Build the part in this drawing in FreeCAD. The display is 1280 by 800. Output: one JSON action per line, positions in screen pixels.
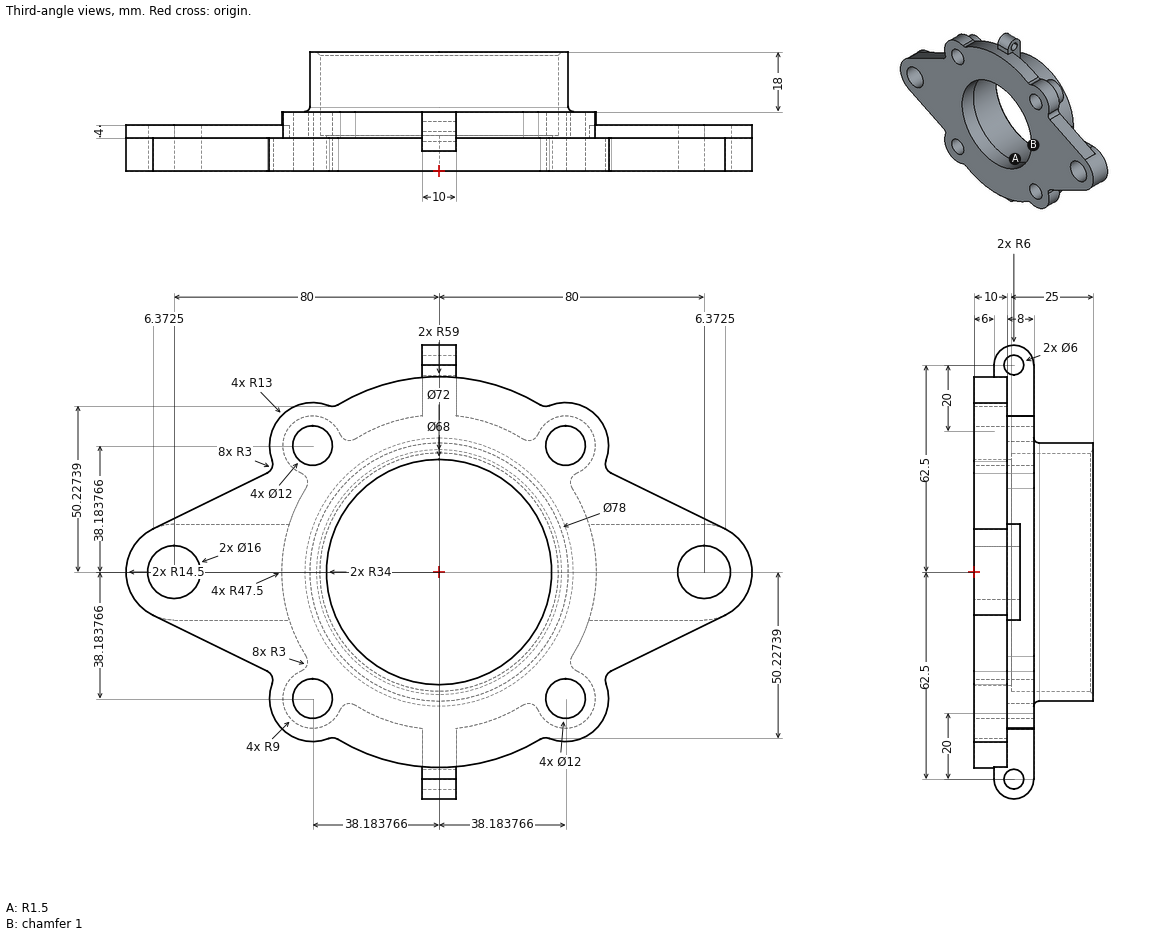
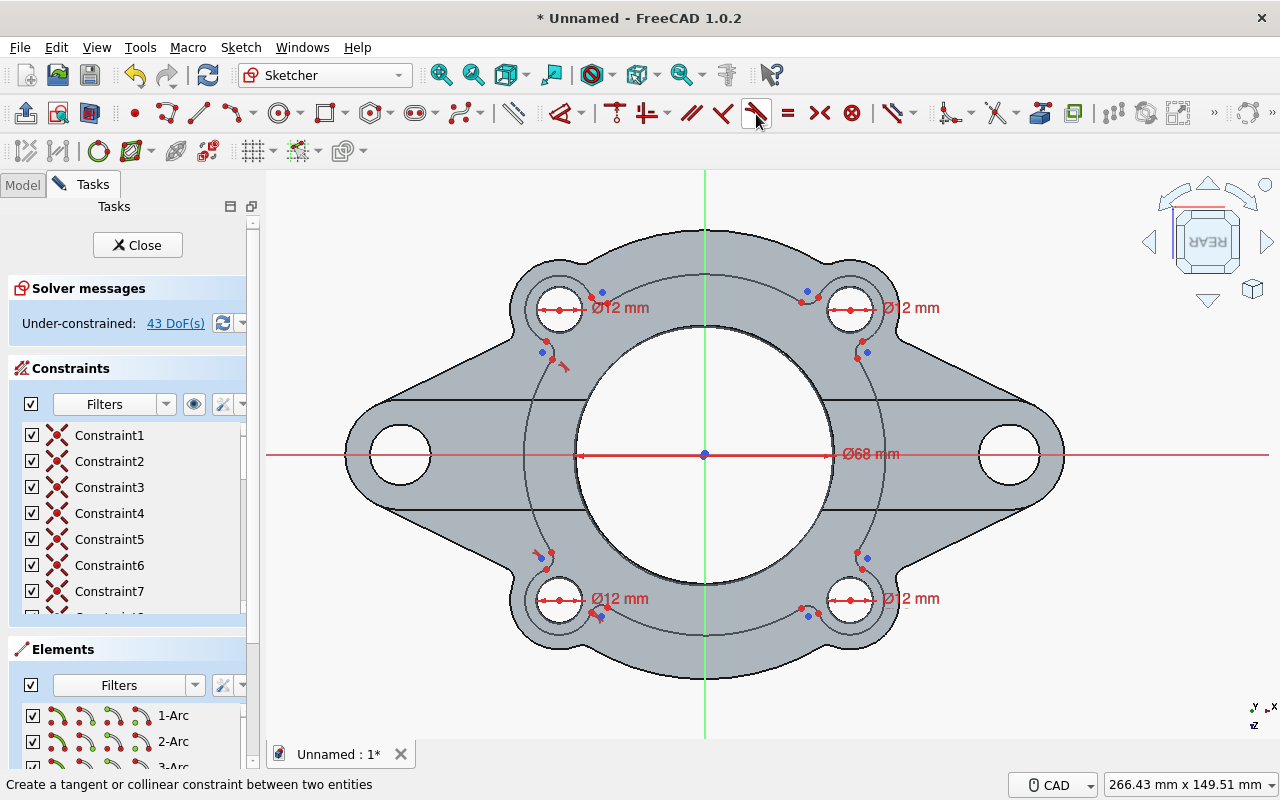
{"action": "left_click", "coordinate": [664, 631]}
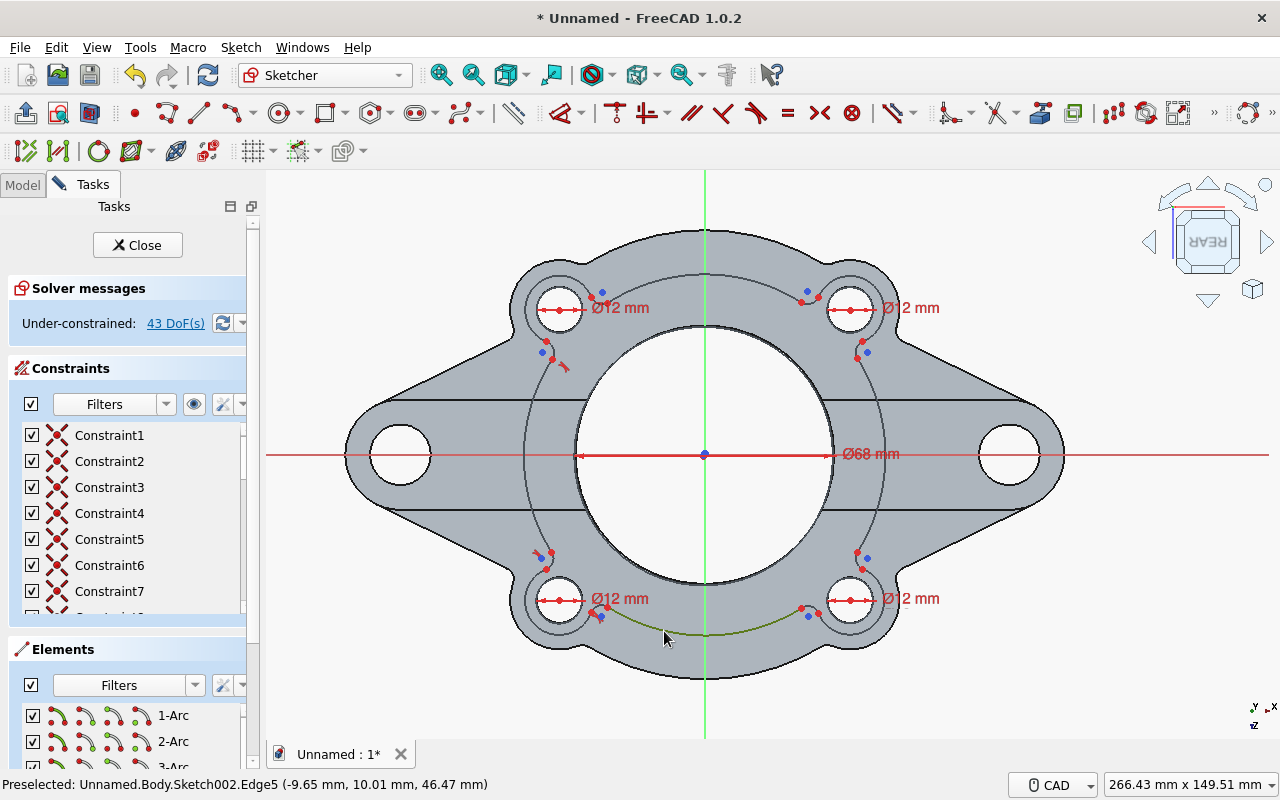
{"action": "scroll", "coordinate": [812, 607], "scroll_direction": "up", "scroll_amount": 2}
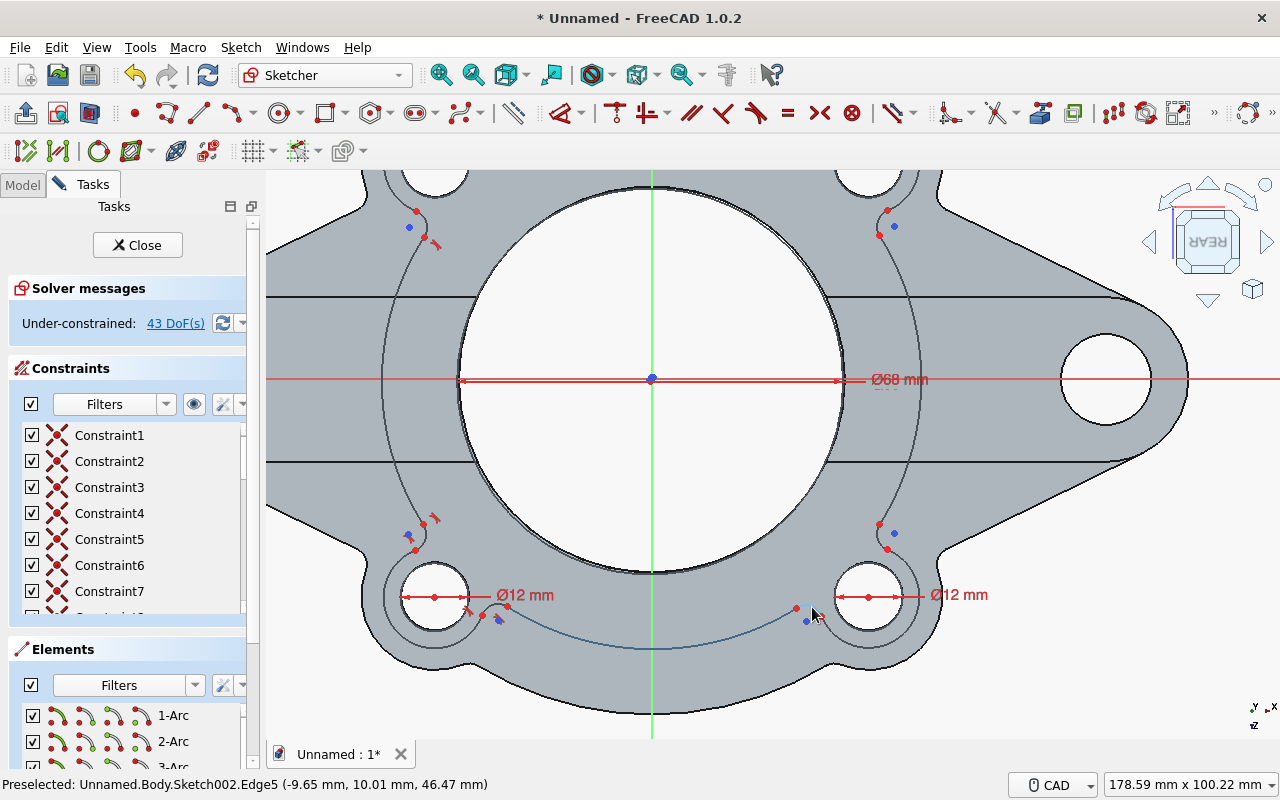
{"action": "left_click", "coordinate": [811, 606]}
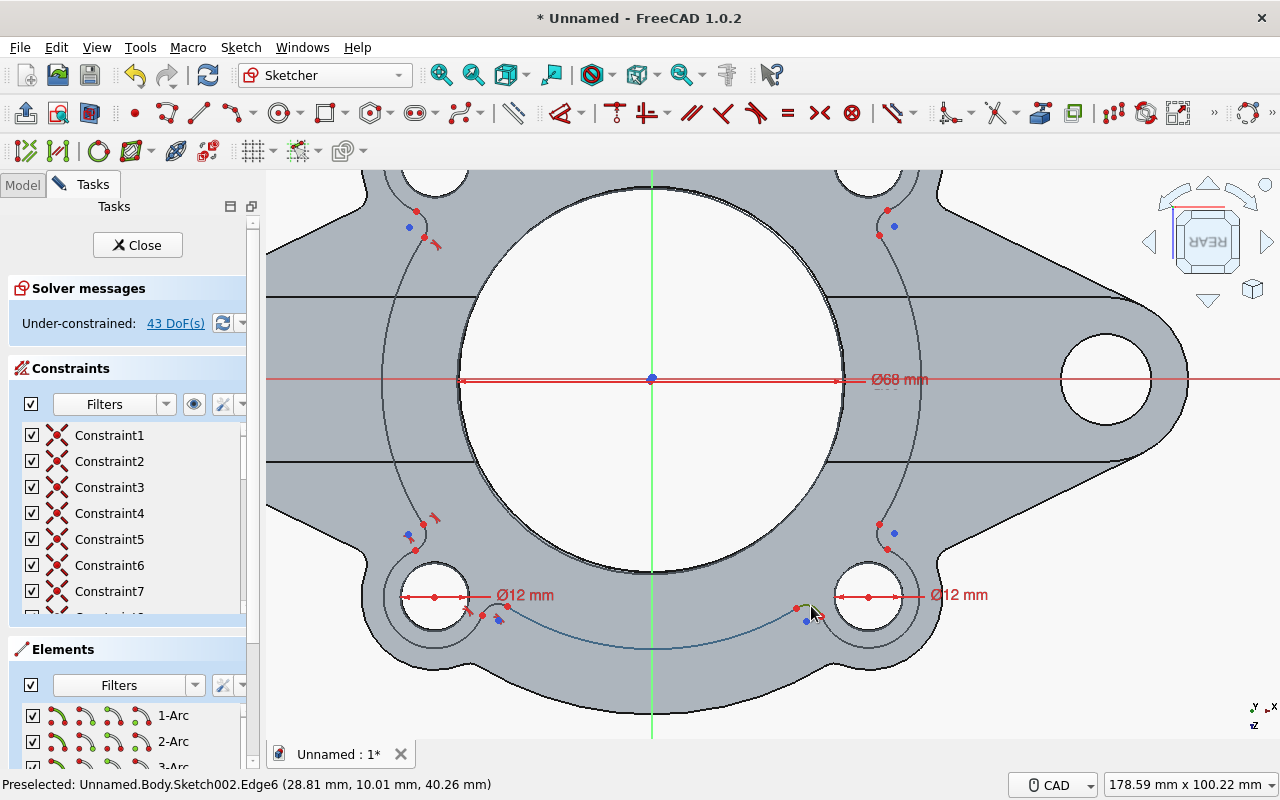
{"action": "left_click", "coordinate": [756, 114]}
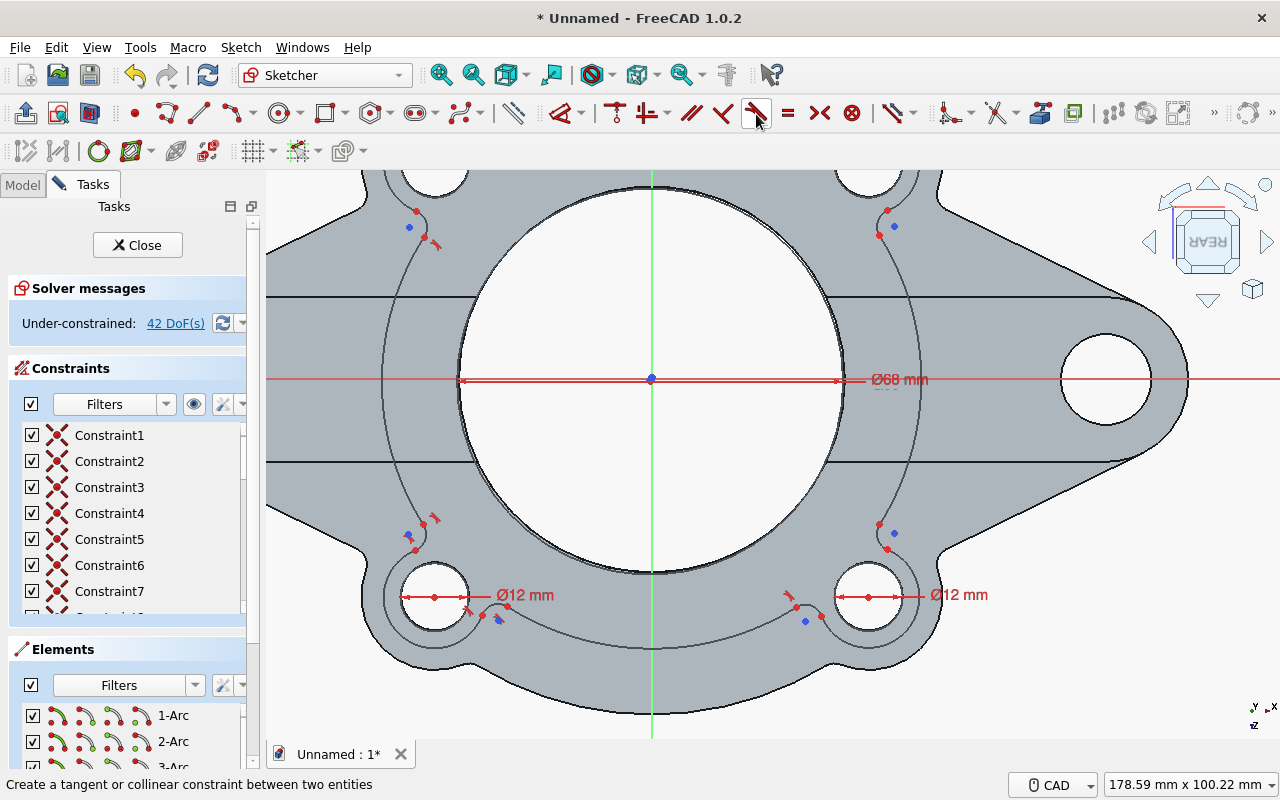
{"action": "scroll", "coordinate": [817, 609], "scroll_direction": "up", "scroll_amount": 3}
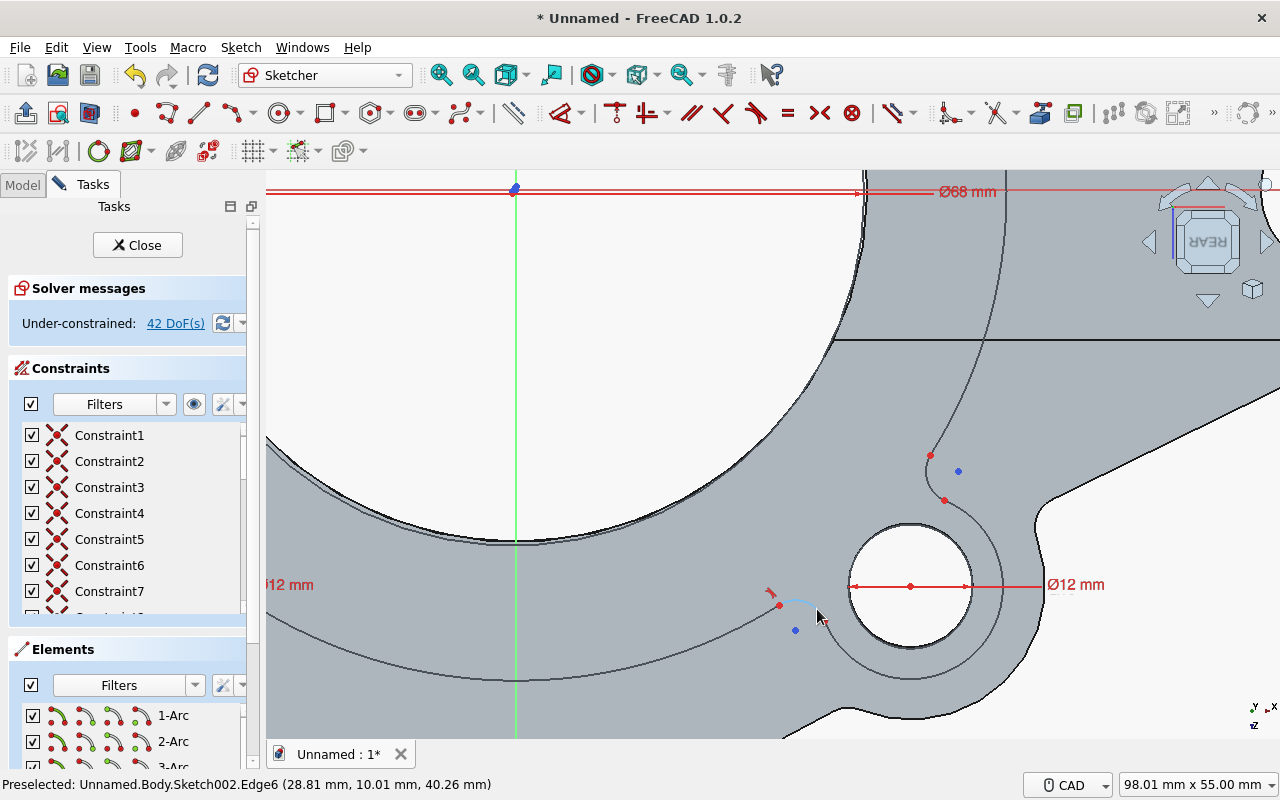
{"action": "left_click", "coordinate": [816, 608]}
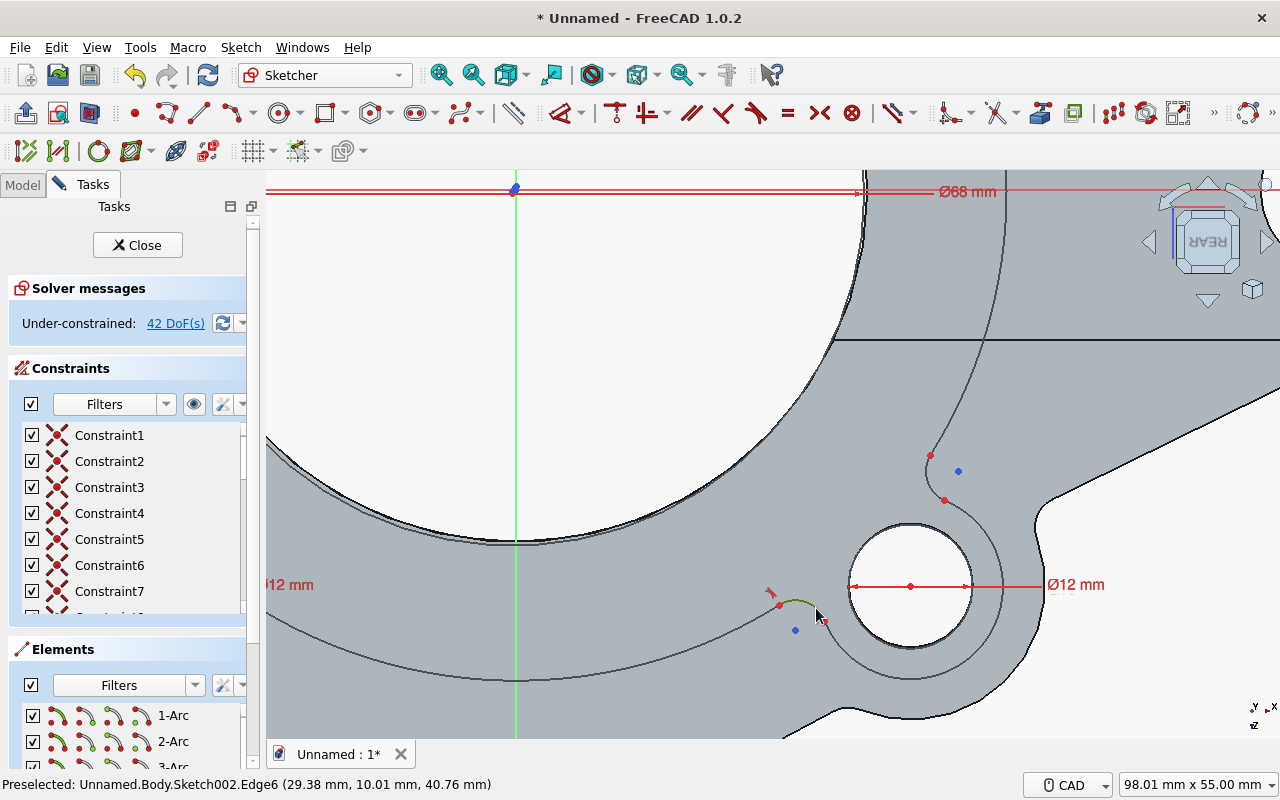
{"action": "left_click", "coordinate": [910, 679]}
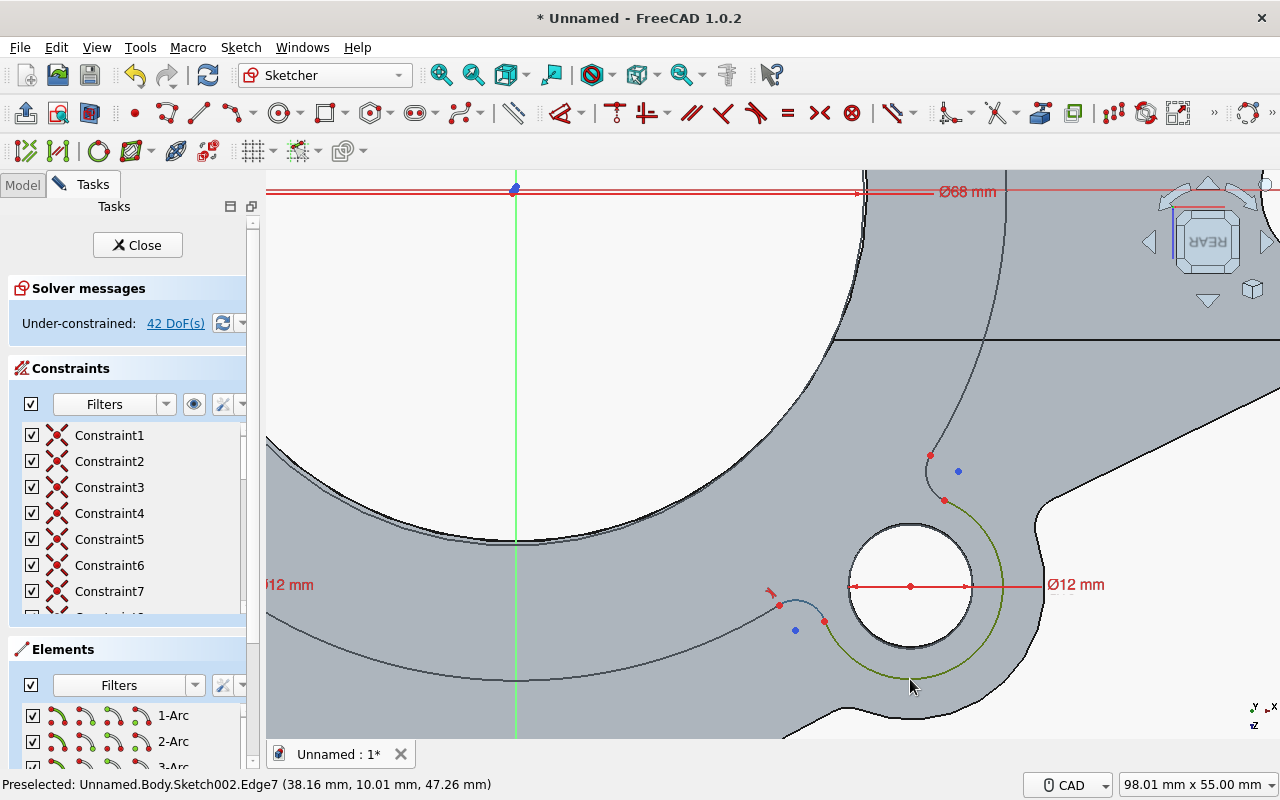
{"action": "left_click", "coordinate": [756, 114]}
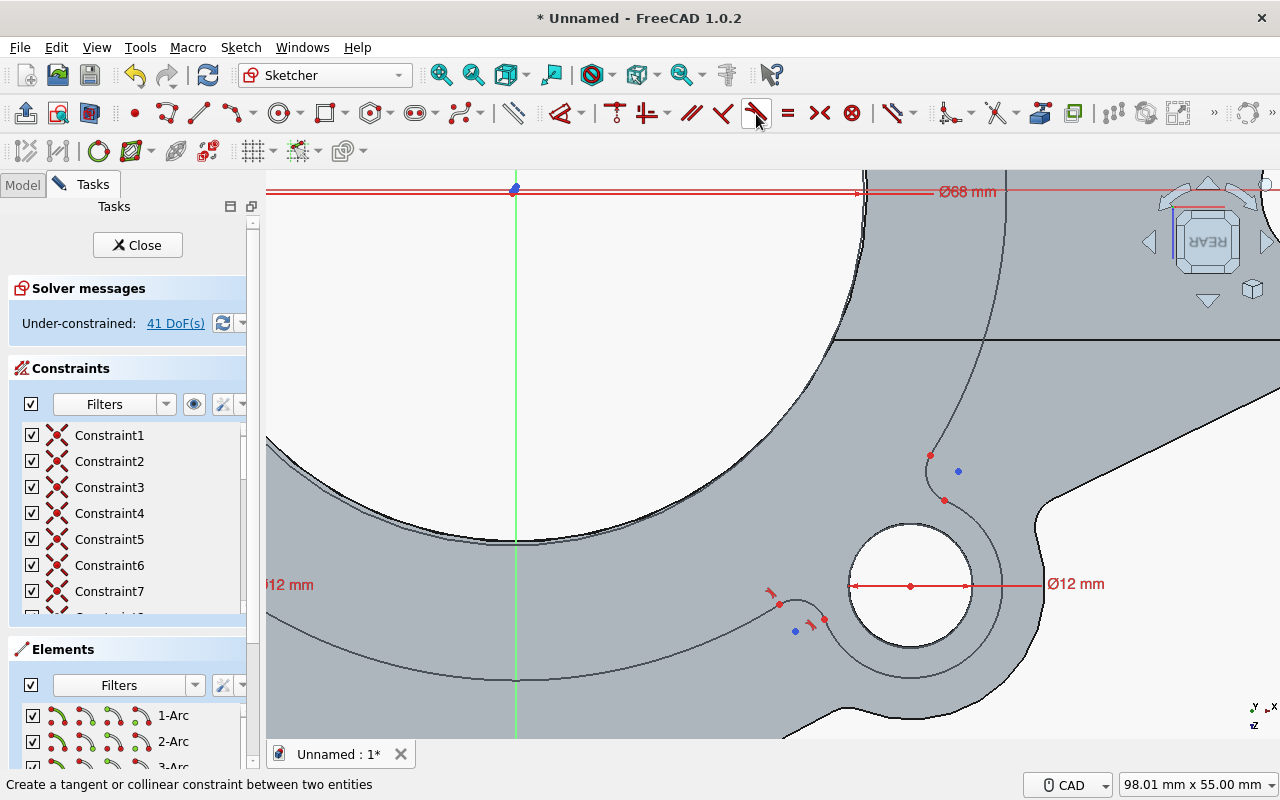
{"action": "left_click", "coordinate": [909, 678]}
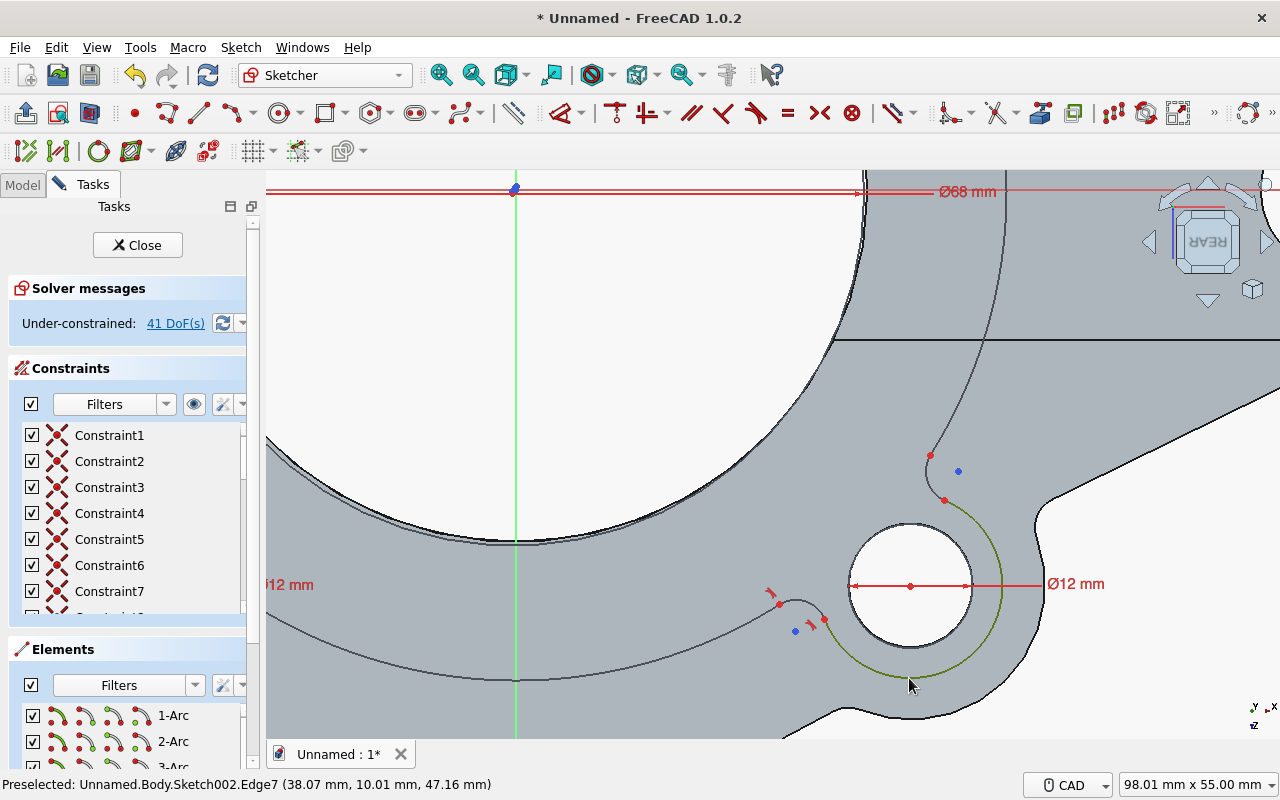
{"action": "left_click", "coordinate": [926, 471]}